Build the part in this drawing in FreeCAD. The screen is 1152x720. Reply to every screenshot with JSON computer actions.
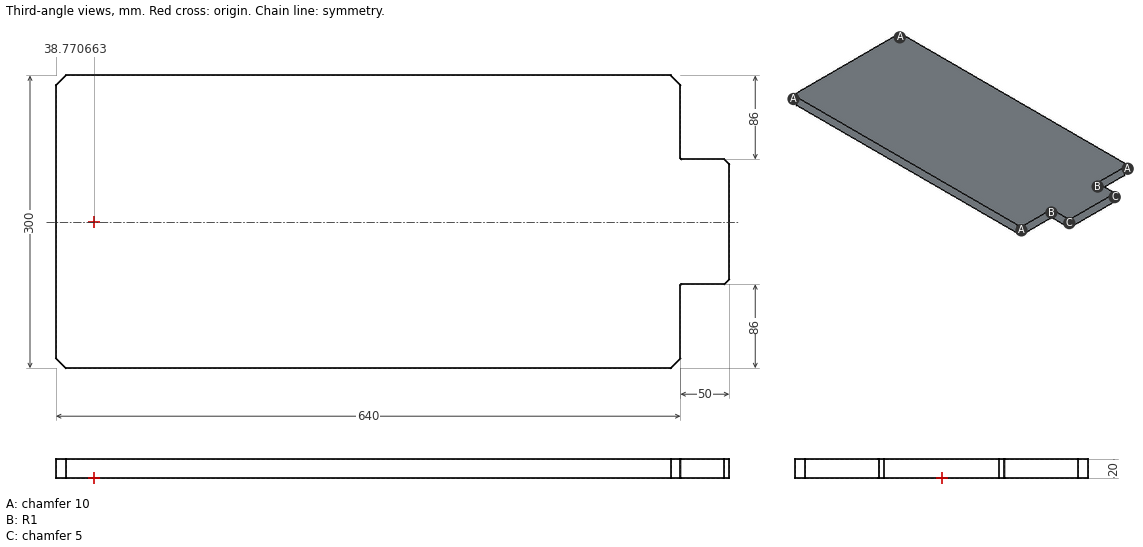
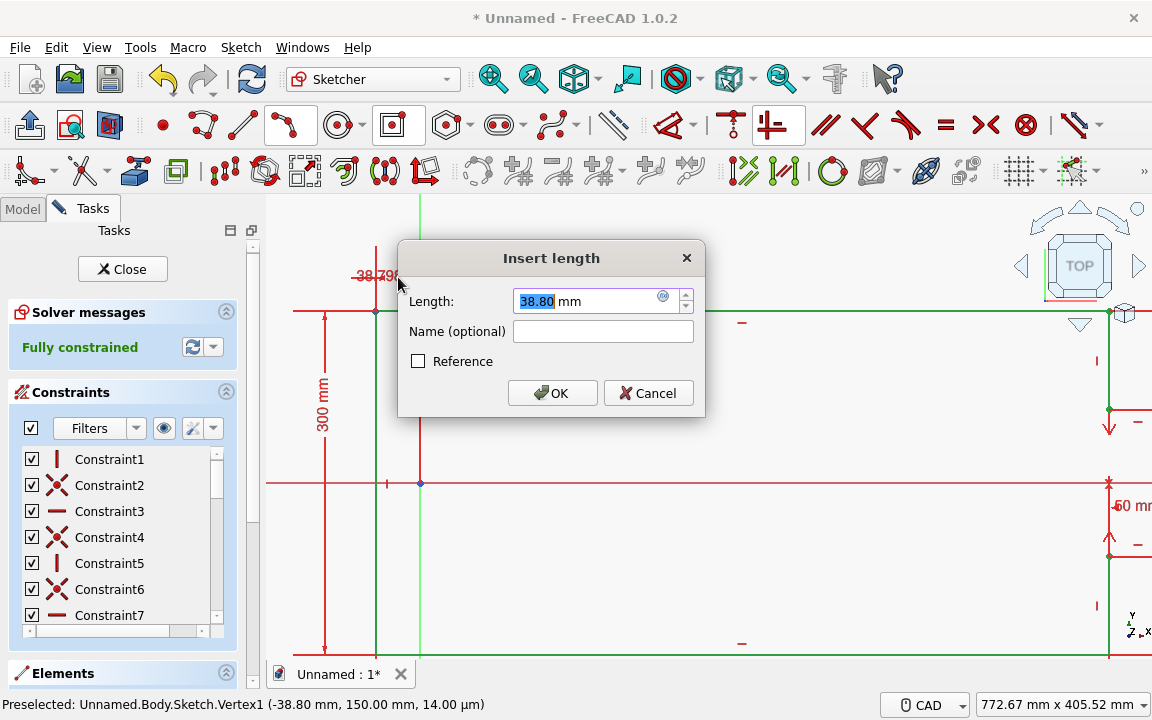
{"action": "type", "text": "38.770663"}
{"action": "key", "text": "Return"}
{"action": "key", "text": "Escape"}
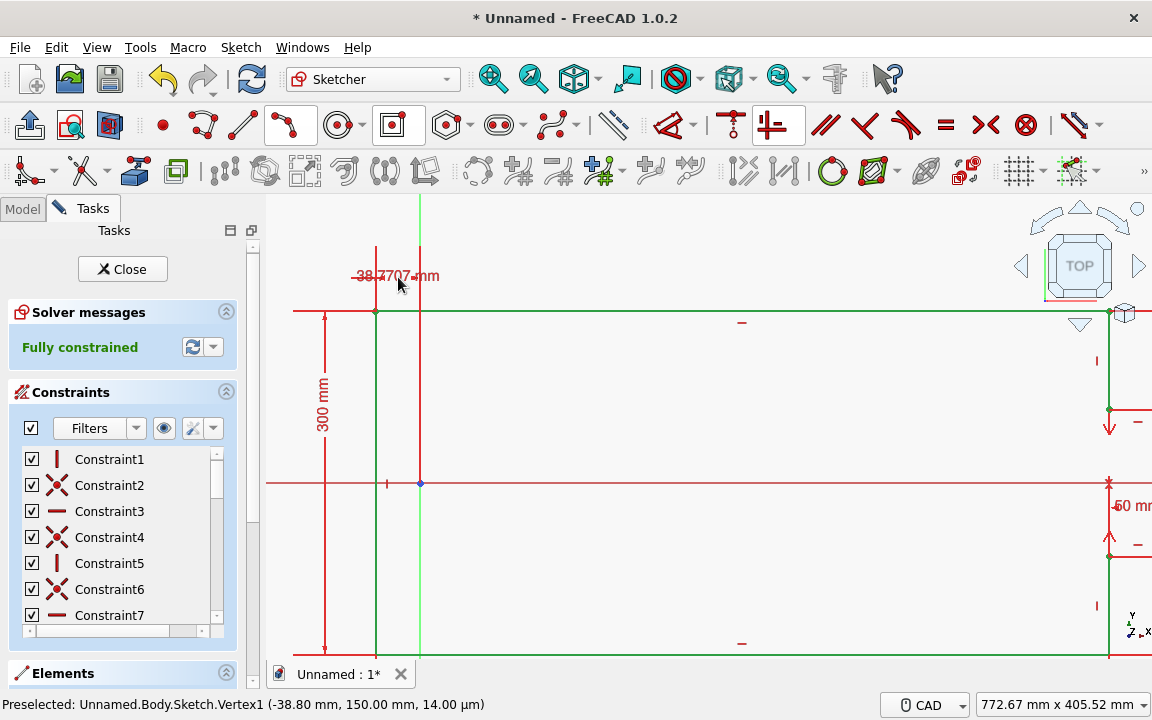
{"action": "left_click", "coordinate": [123, 269]}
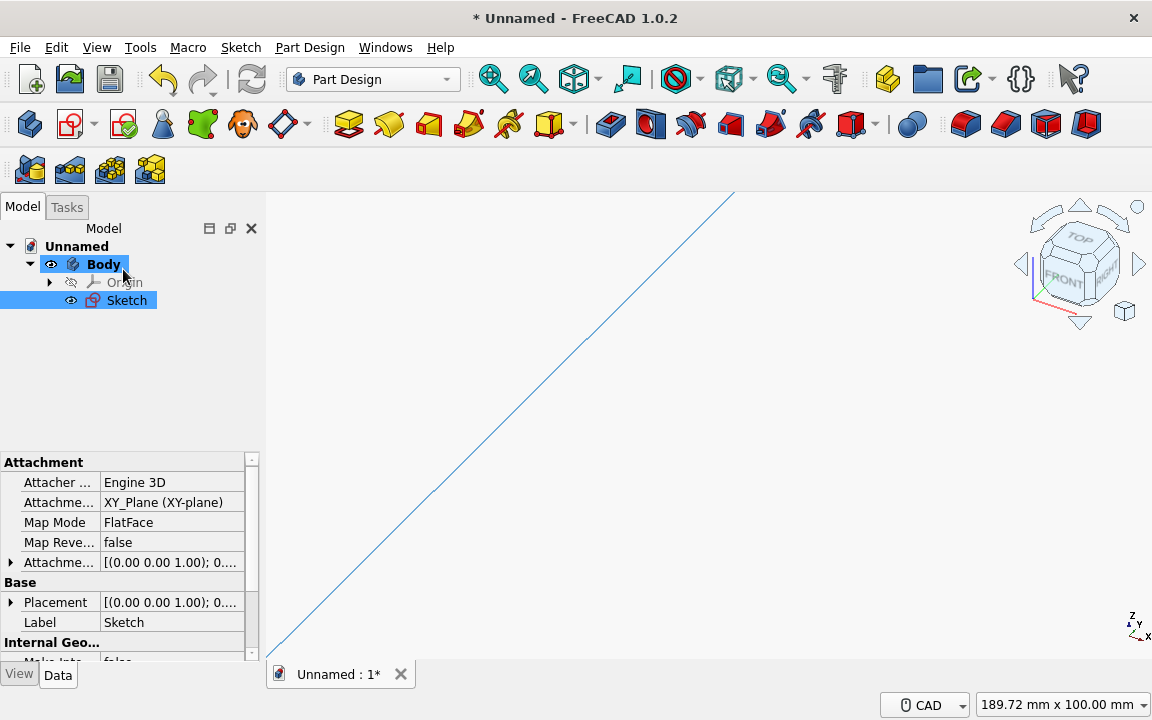
{"action": "left_click", "coordinate": [350, 124]}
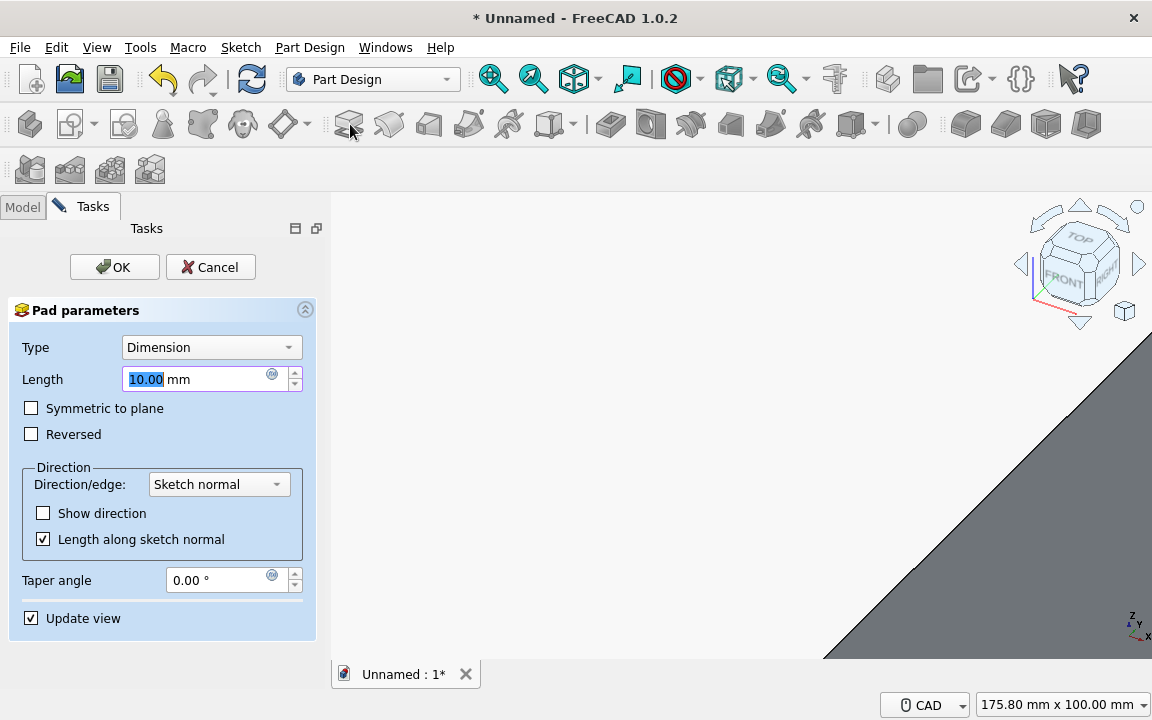
{"action": "type", "text": "20"}
{"action": "key", "text": "Tab"}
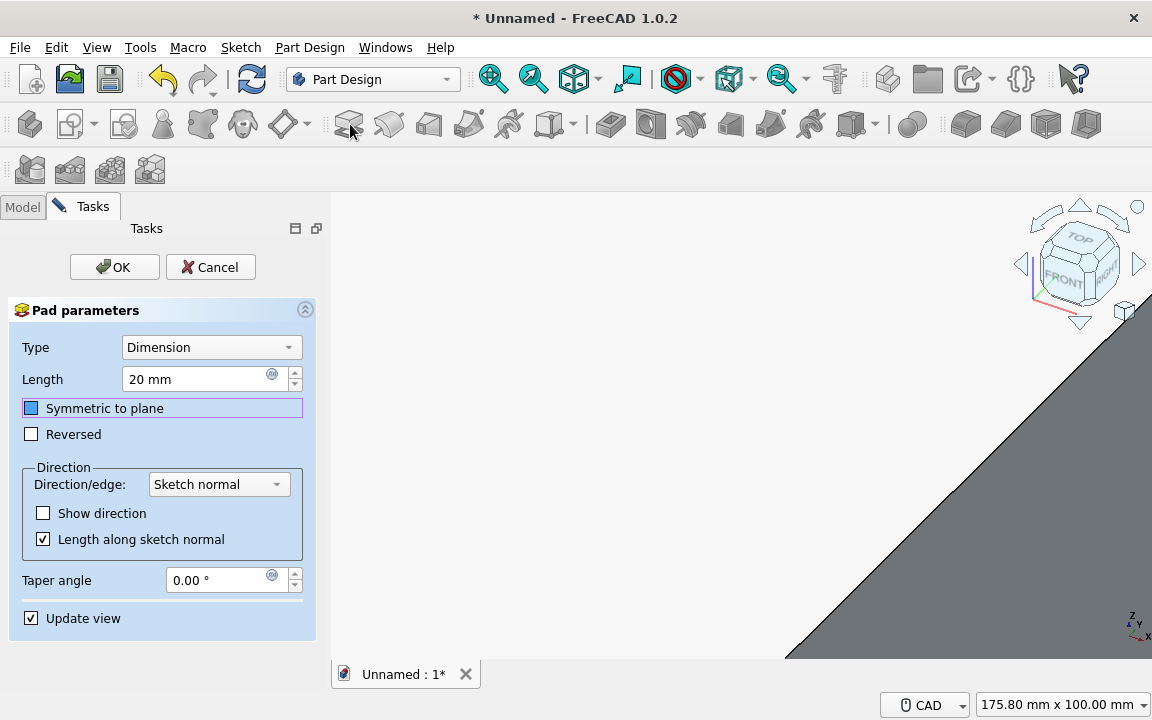
{"action": "left_click", "coordinate": [115, 267]}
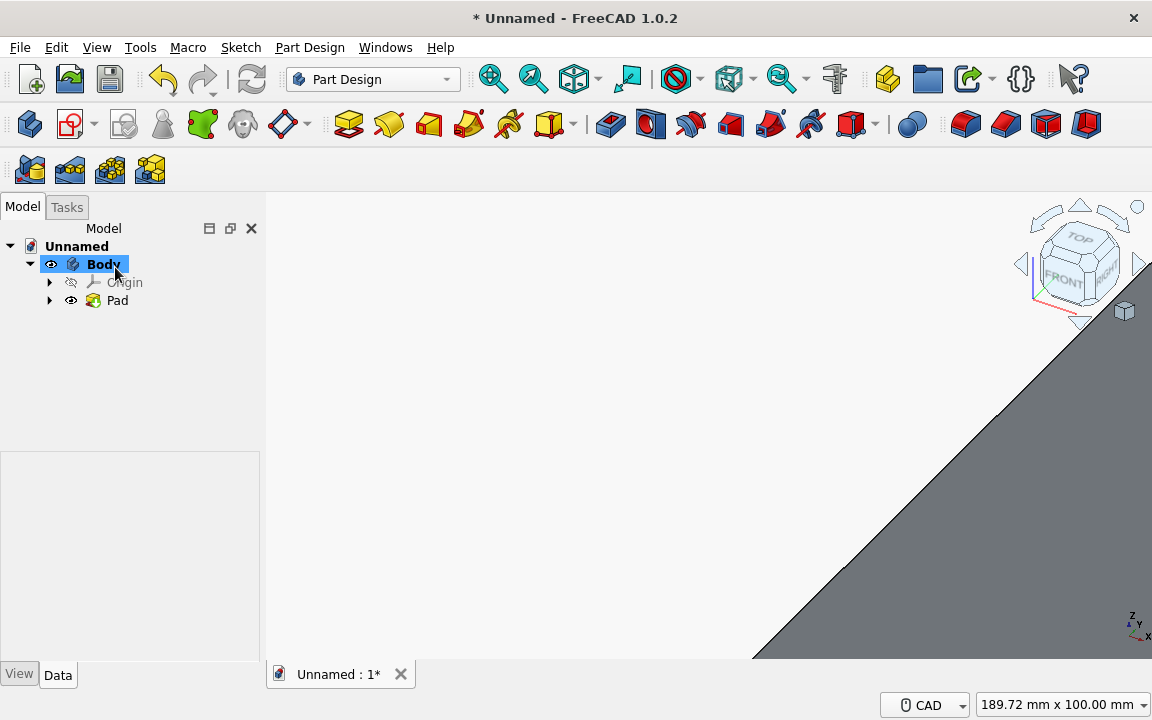
{"action": "left_click", "coordinate": [494, 80]}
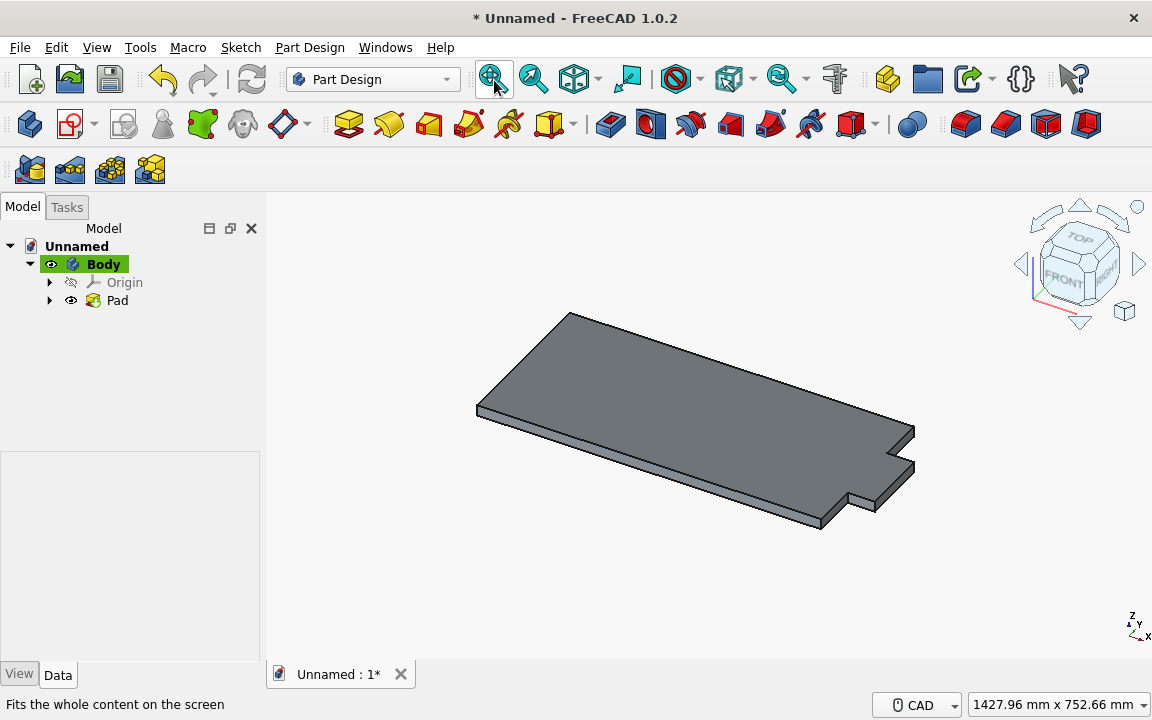
{"action": "left_click", "coordinate": [821, 525]}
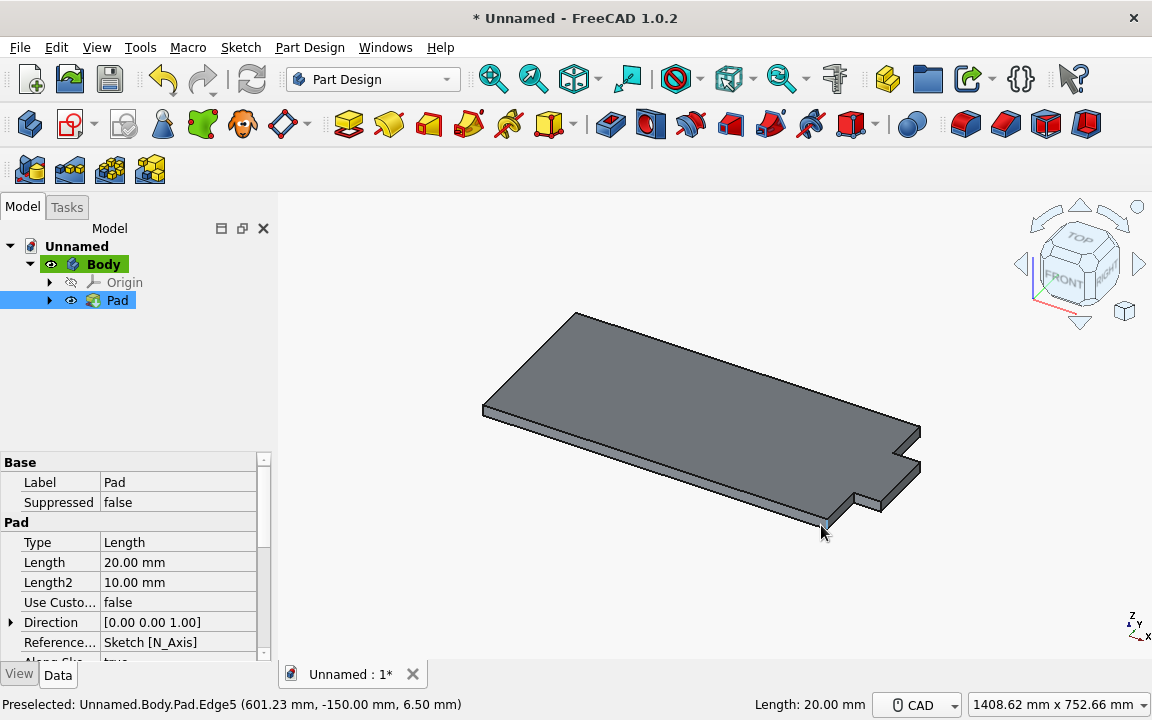
{"action": "scroll", "coordinate": [920, 431], "scroll_direction": "up", "scroll_amount": 6}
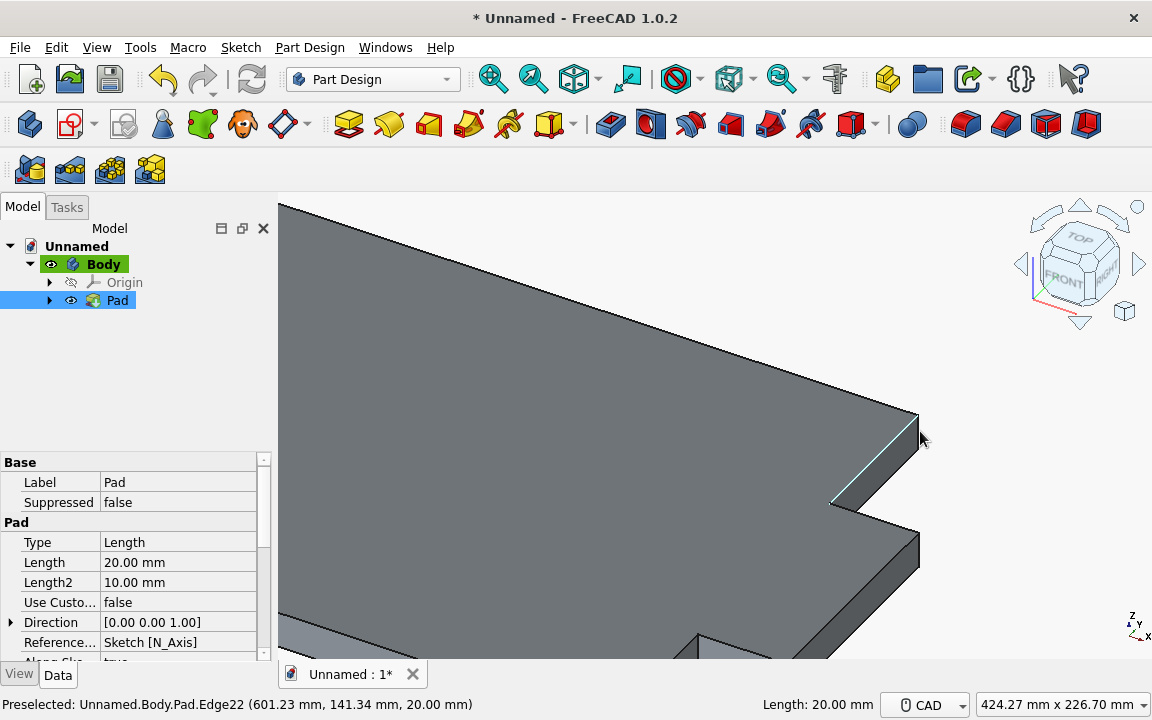
{"action": "left_click", "coordinate": [494, 80]}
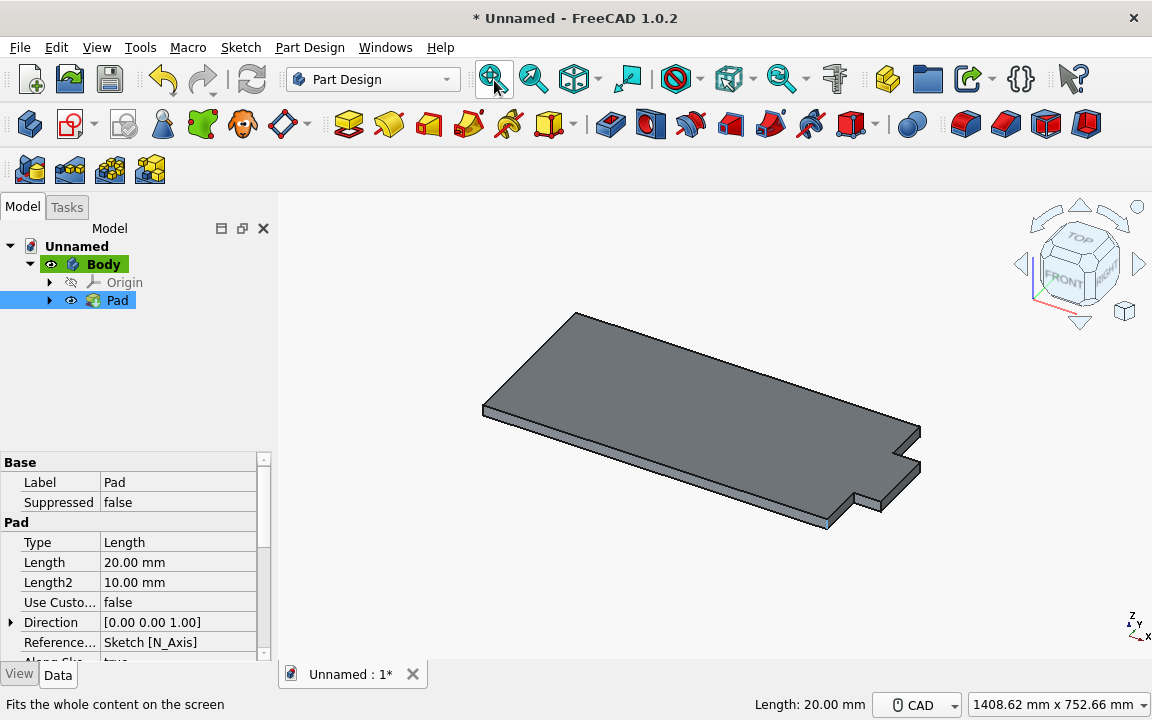
{"action": "key", "text": "0"}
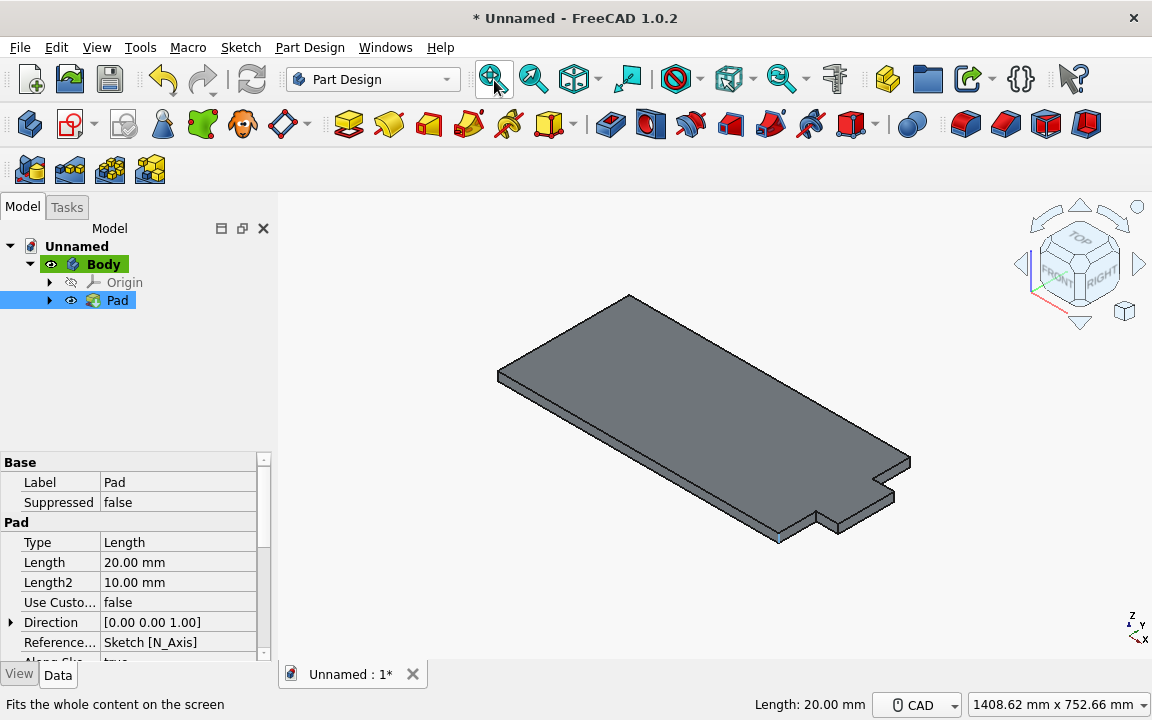
{"action": "scroll", "coordinate": [910, 461], "scroll_direction": "up", "scroll_amount": 6}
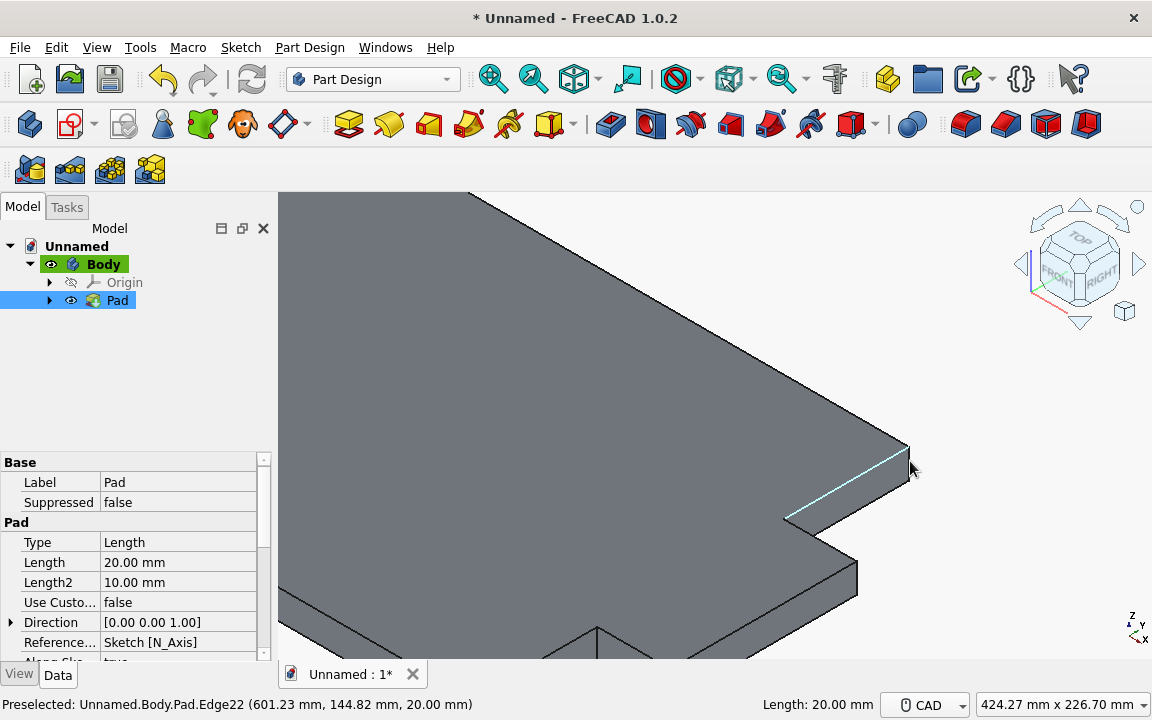
{"action": "left_click", "coordinate": [494, 80]}